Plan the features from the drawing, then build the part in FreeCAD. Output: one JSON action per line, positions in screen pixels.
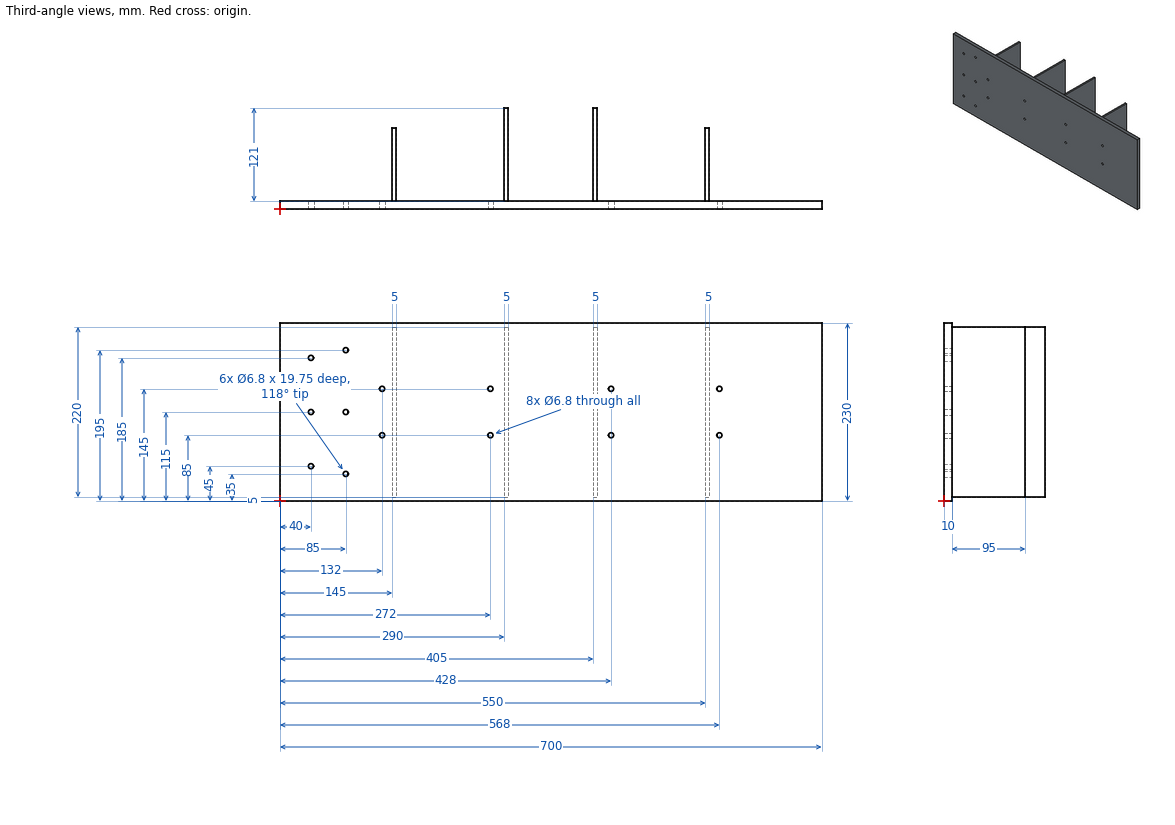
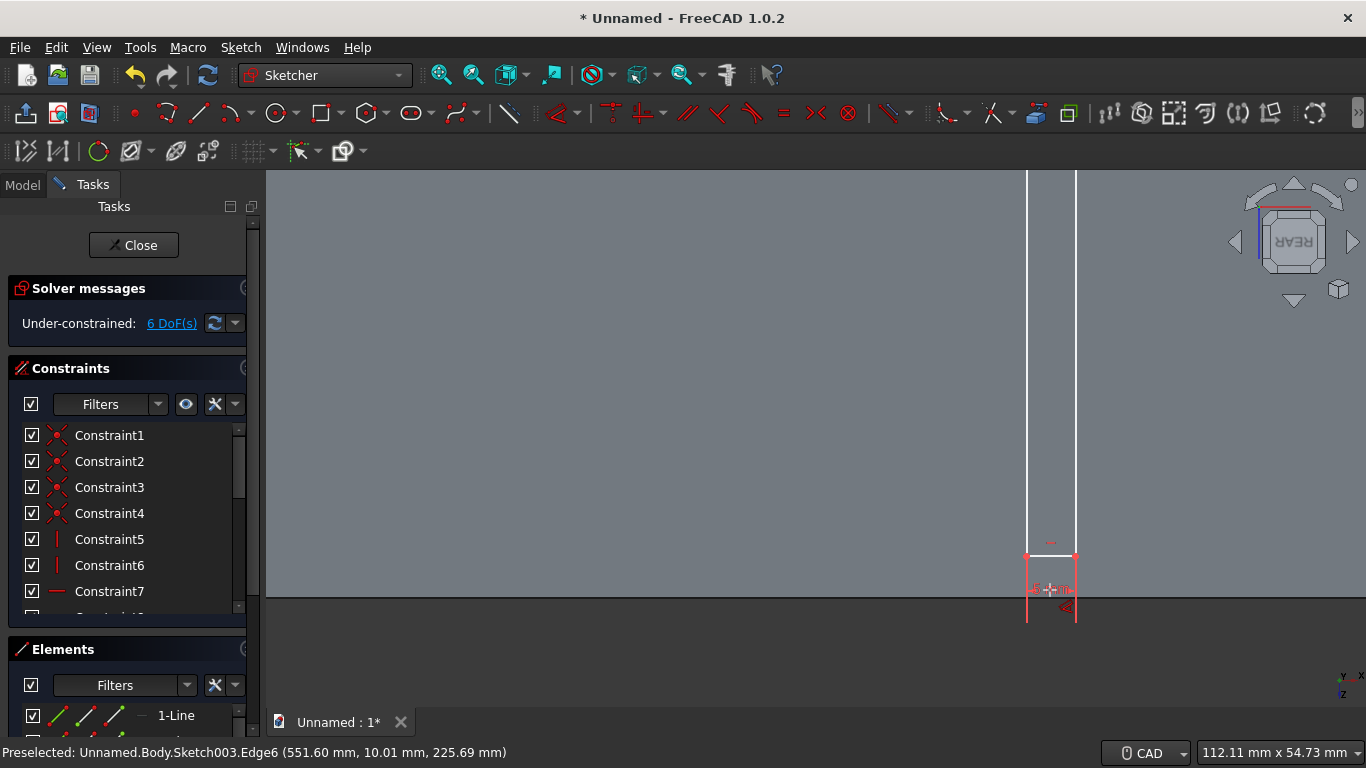
{"action": "scroll", "coordinate": [1046, 562], "scroll_direction": "down", "scroll_amount": 11}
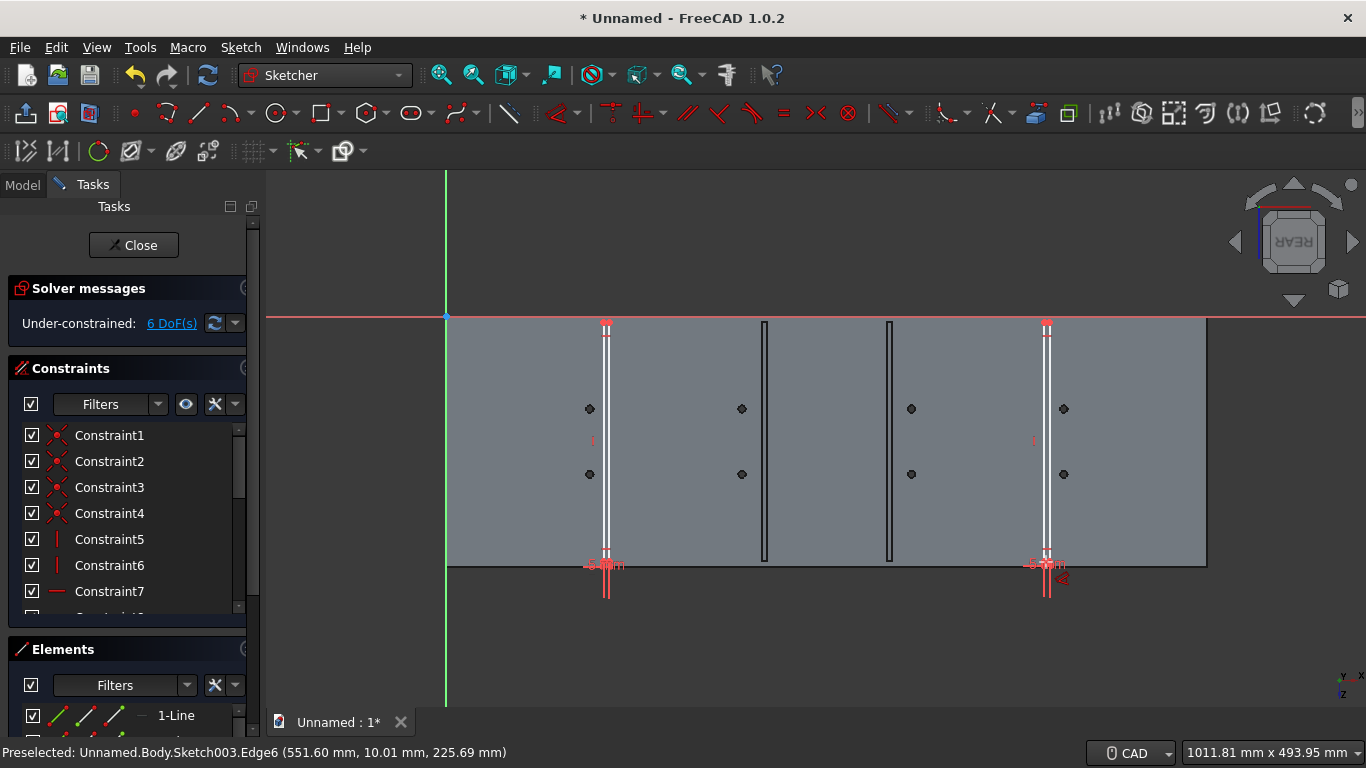
{"action": "scroll", "coordinate": [604, 322], "scroll_direction": "up", "scroll_amount": 10}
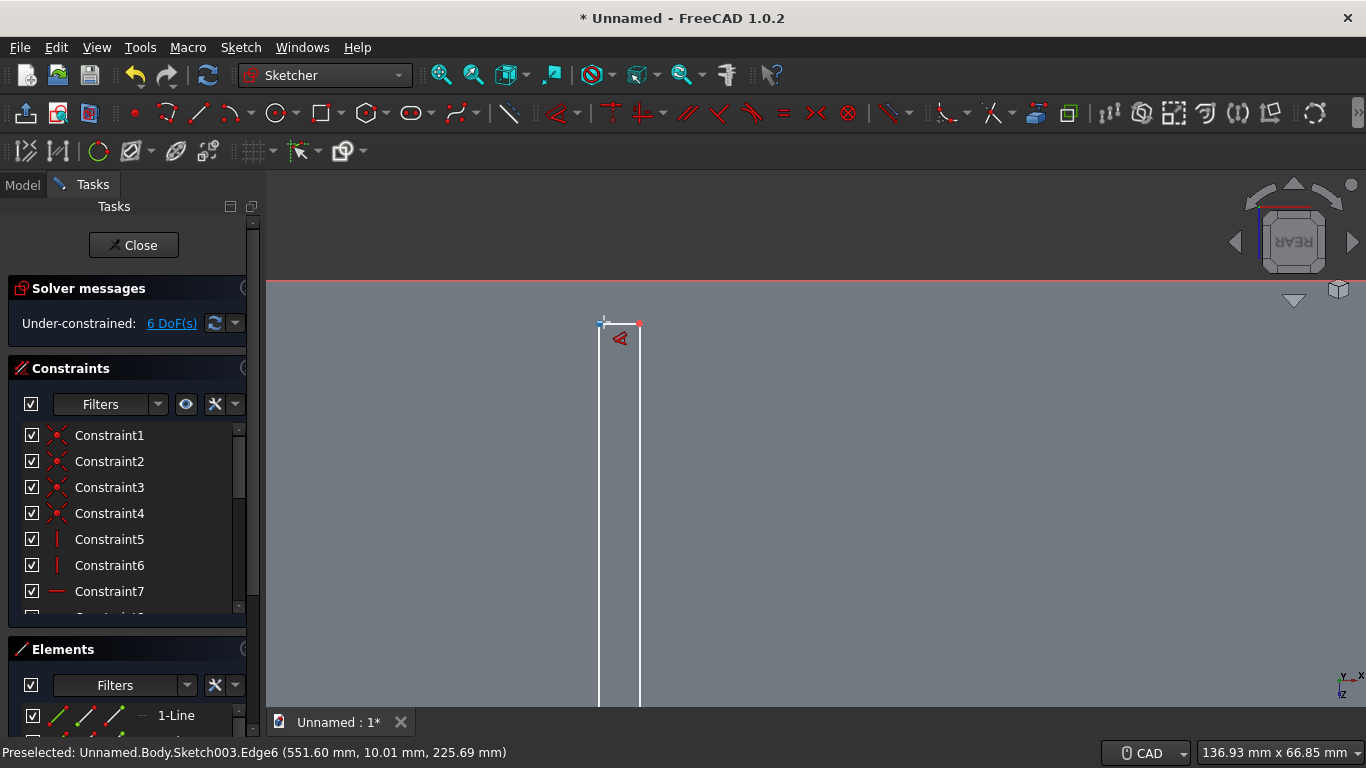
{"action": "left_click", "coordinate": [599, 324]}
{"action": "left_click", "coordinate": [633, 302]}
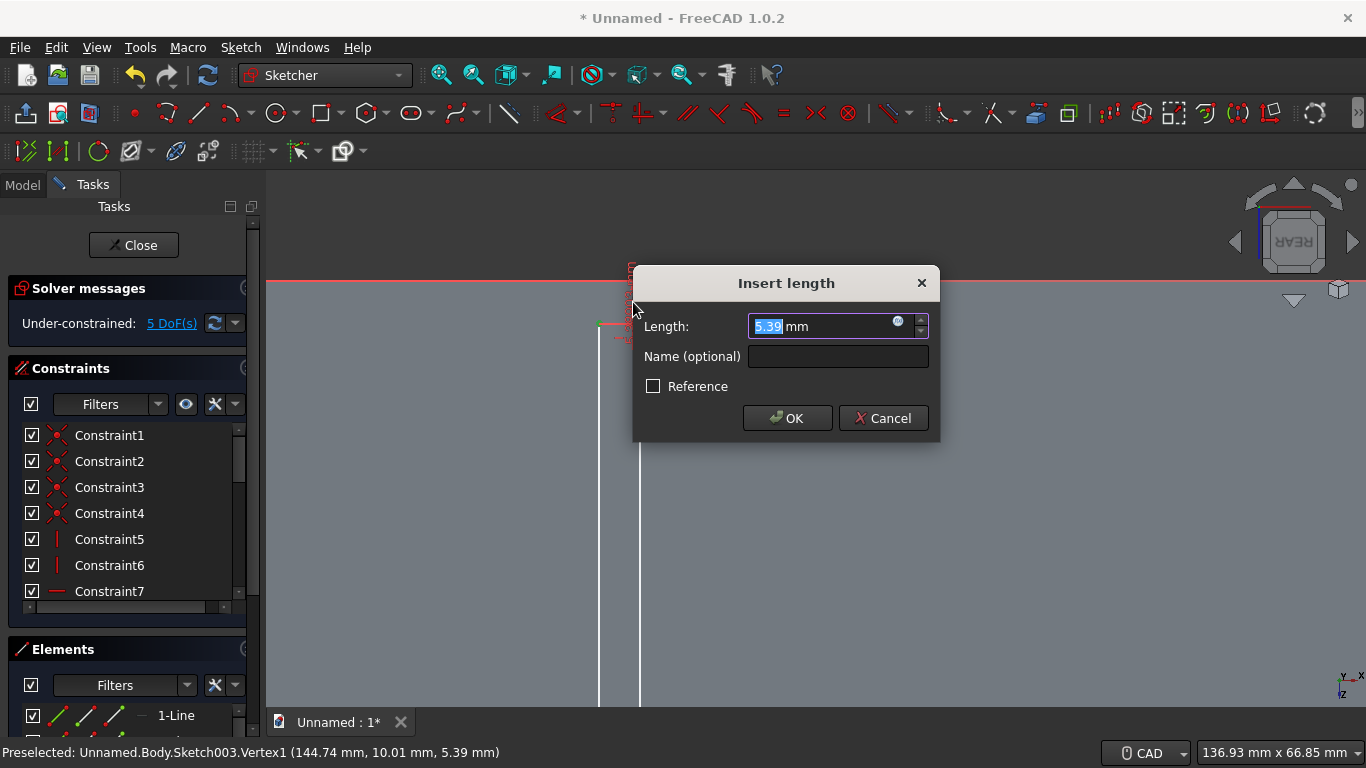
{"action": "type", "text": "5"}
{"action": "key", "text": "Return"}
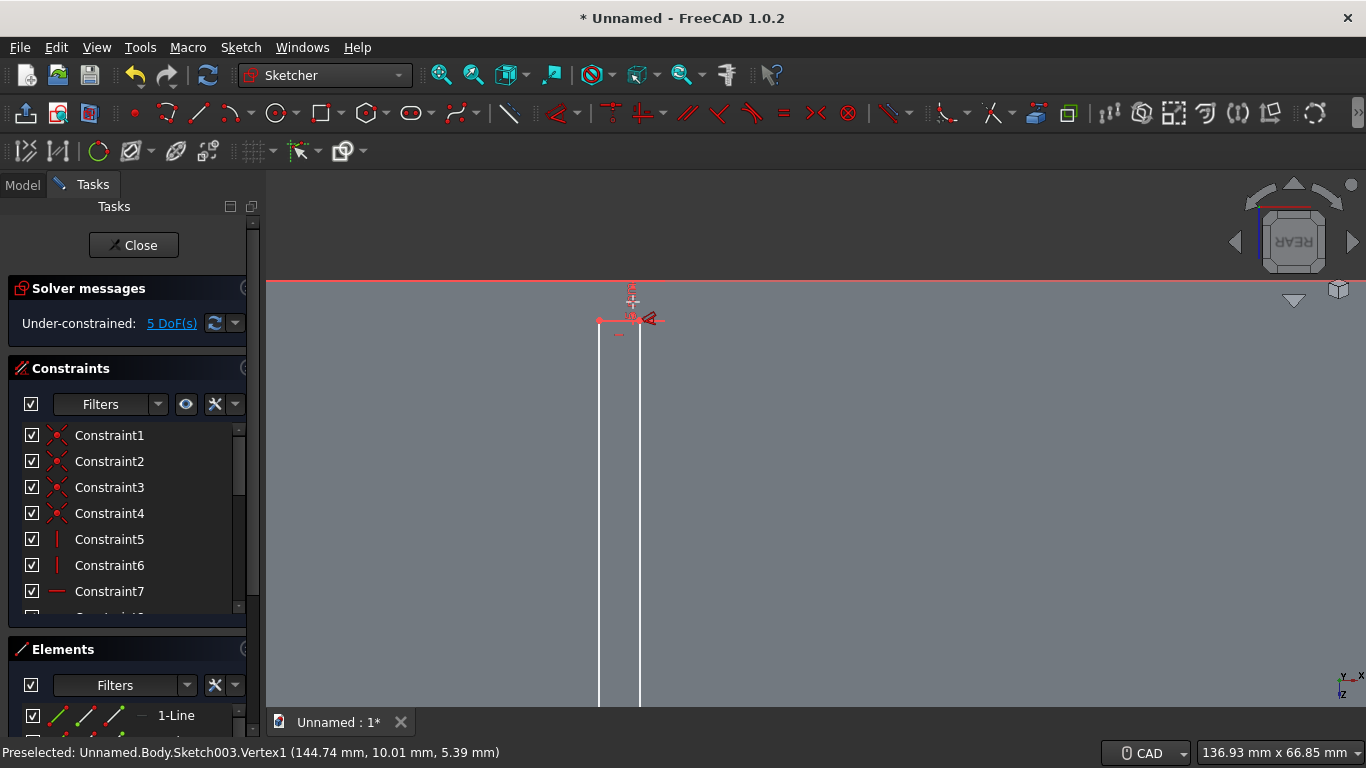
{"action": "scroll", "coordinate": [604, 322], "scroll_direction": "down", "scroll_amount": 10}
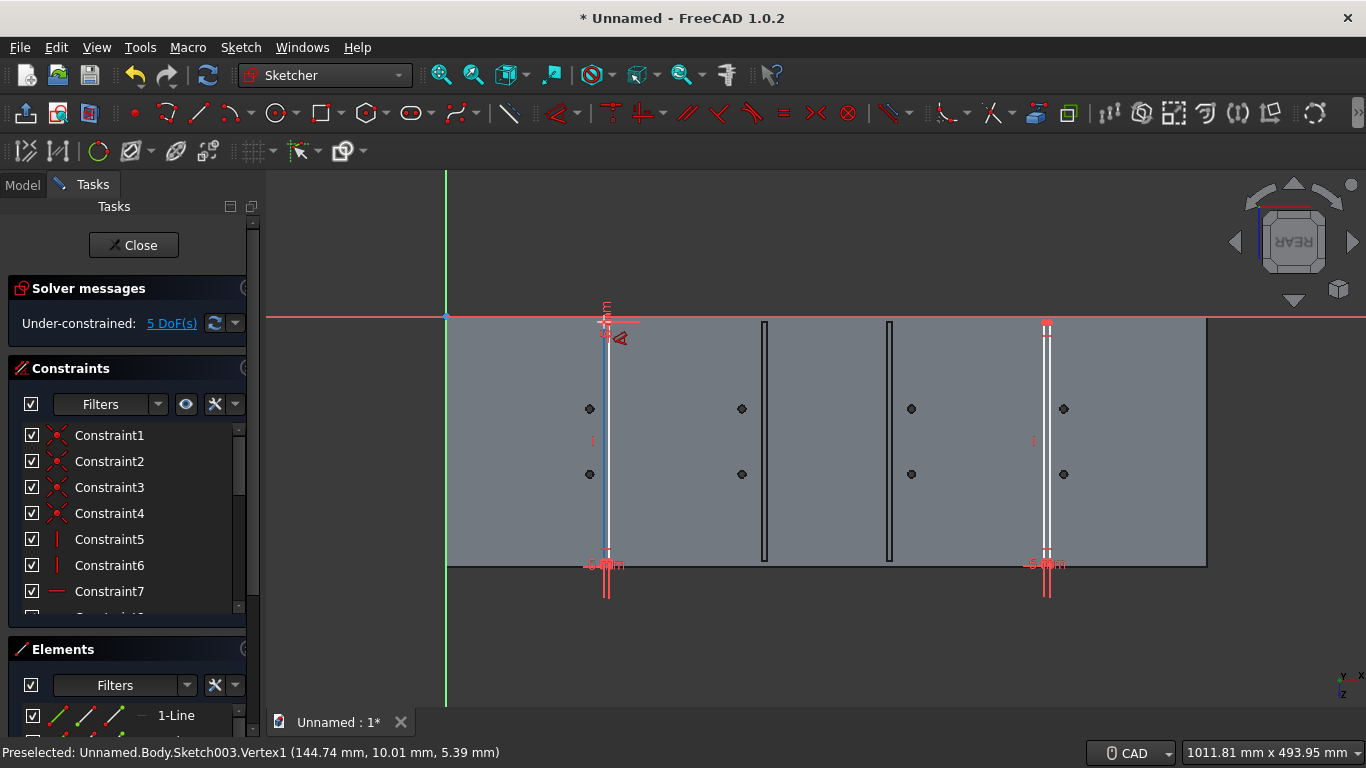
{"action": "scroll", "coordinate": [1044, 322], "scroll_direction": "up", "scroll_amount": 10}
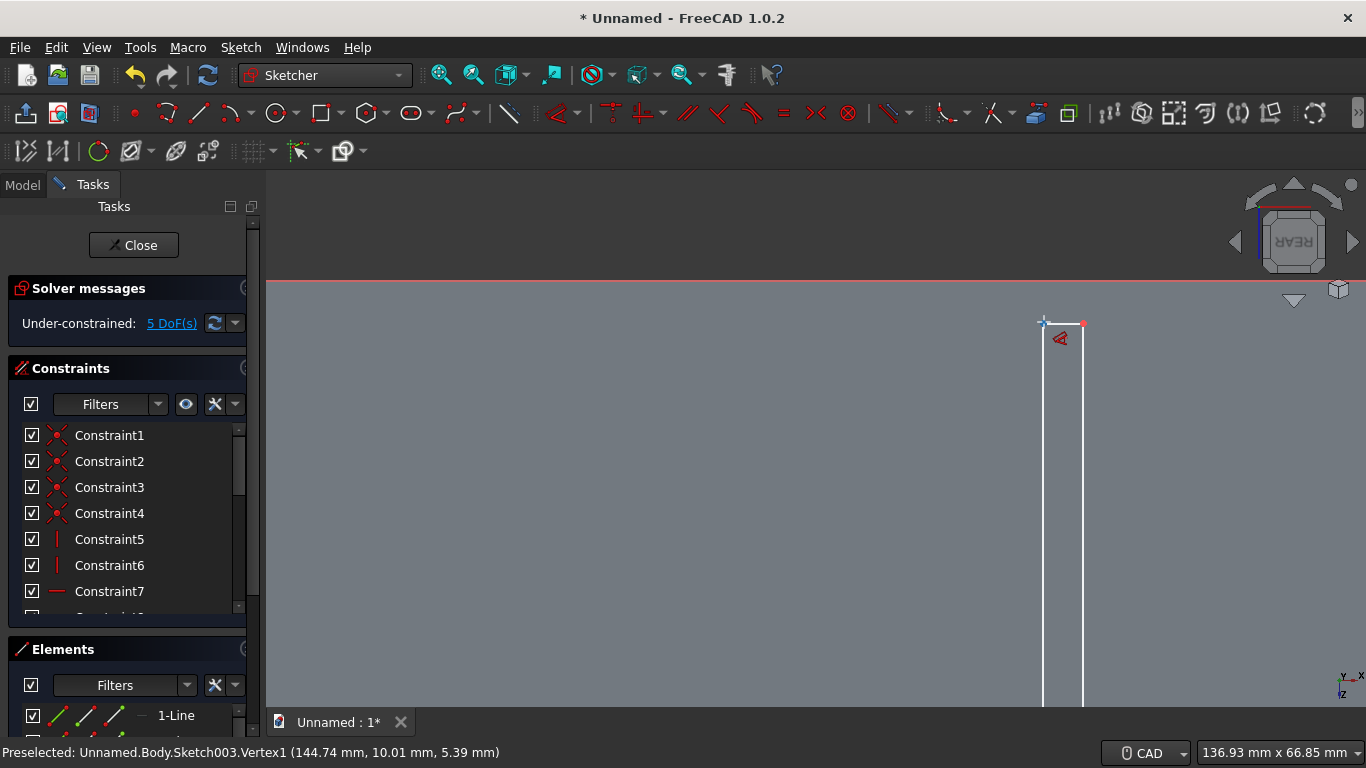
{"action": "left_click", "coordinate": [1043, 324]}
{"action": "left_click", "coordinate": [1077, 302]}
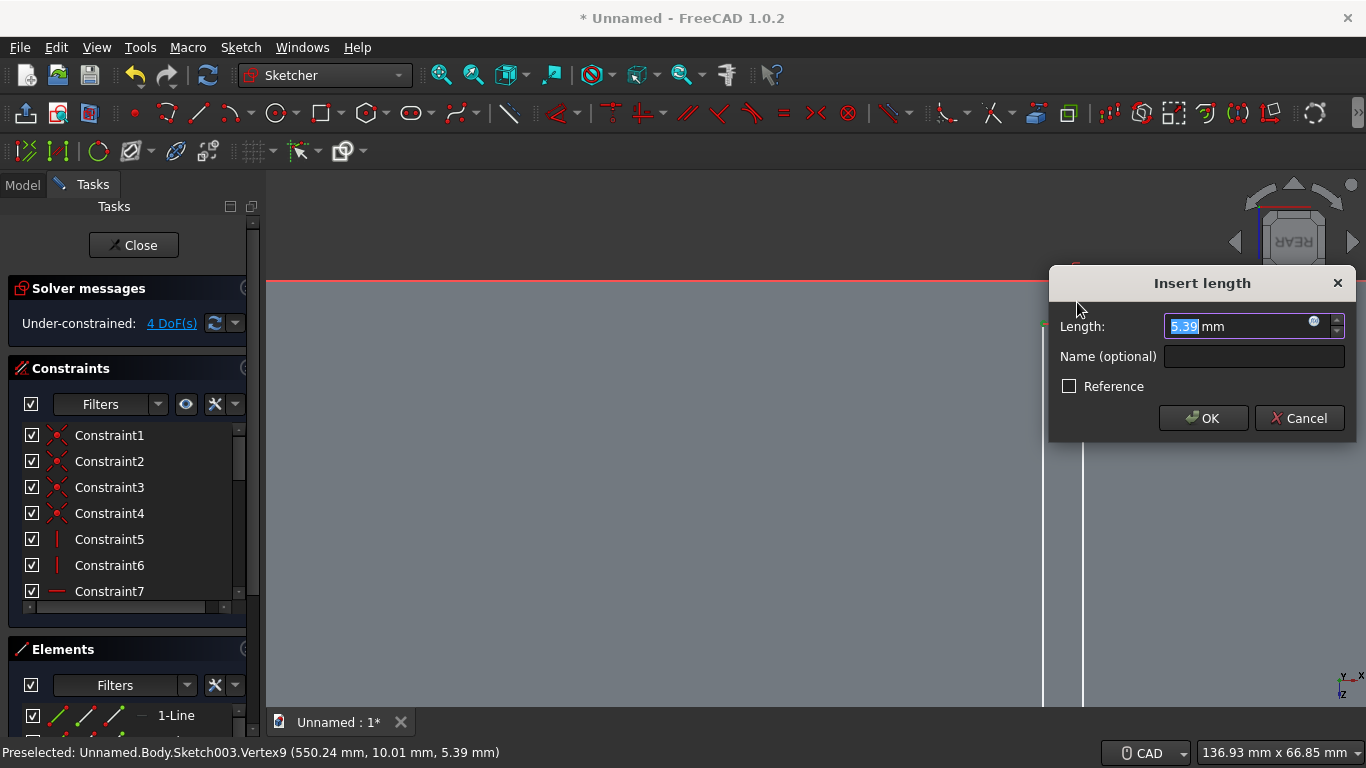
{"action": "type", "text": "5"}
{"action": "key", "text": "Return"}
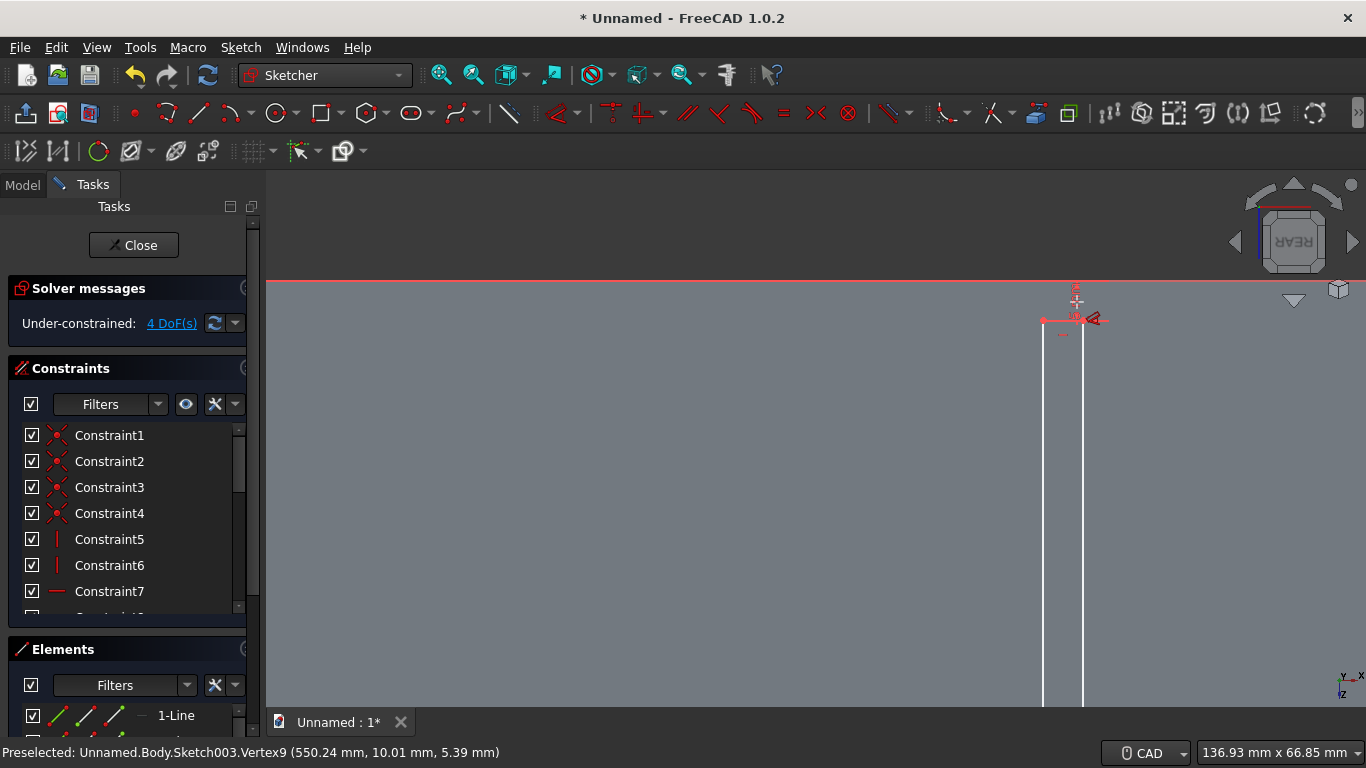
{"action": "scroll", "coordinate": [1044, 322], "scroll_direction": "down", "scroll_amount": 10}